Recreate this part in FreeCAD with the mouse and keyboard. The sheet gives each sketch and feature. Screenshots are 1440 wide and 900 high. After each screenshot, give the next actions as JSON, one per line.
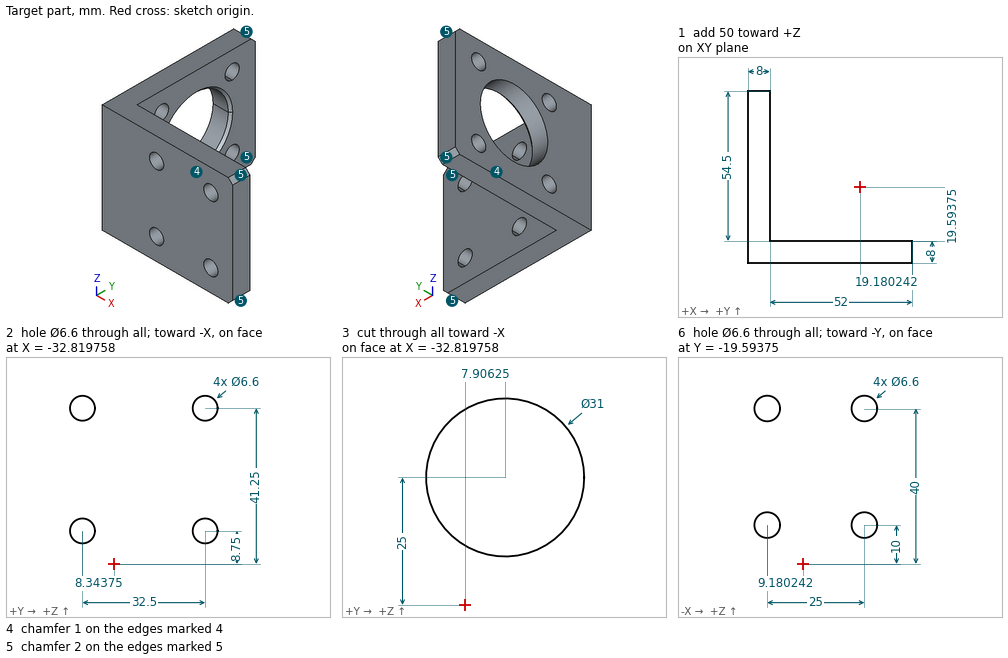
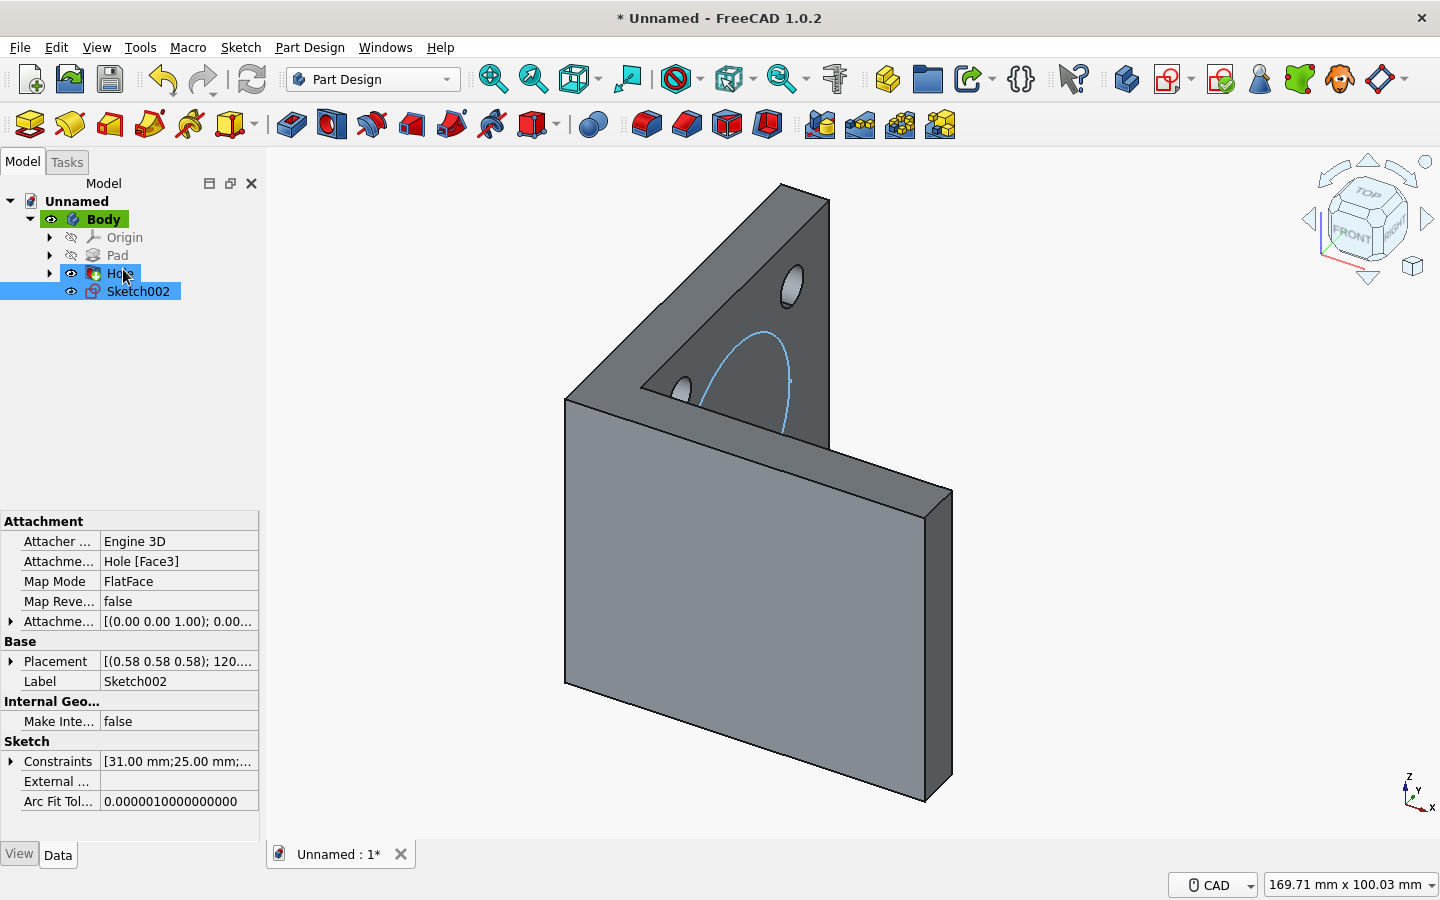
{"action": "left_click", "coordinate": [292, 124]}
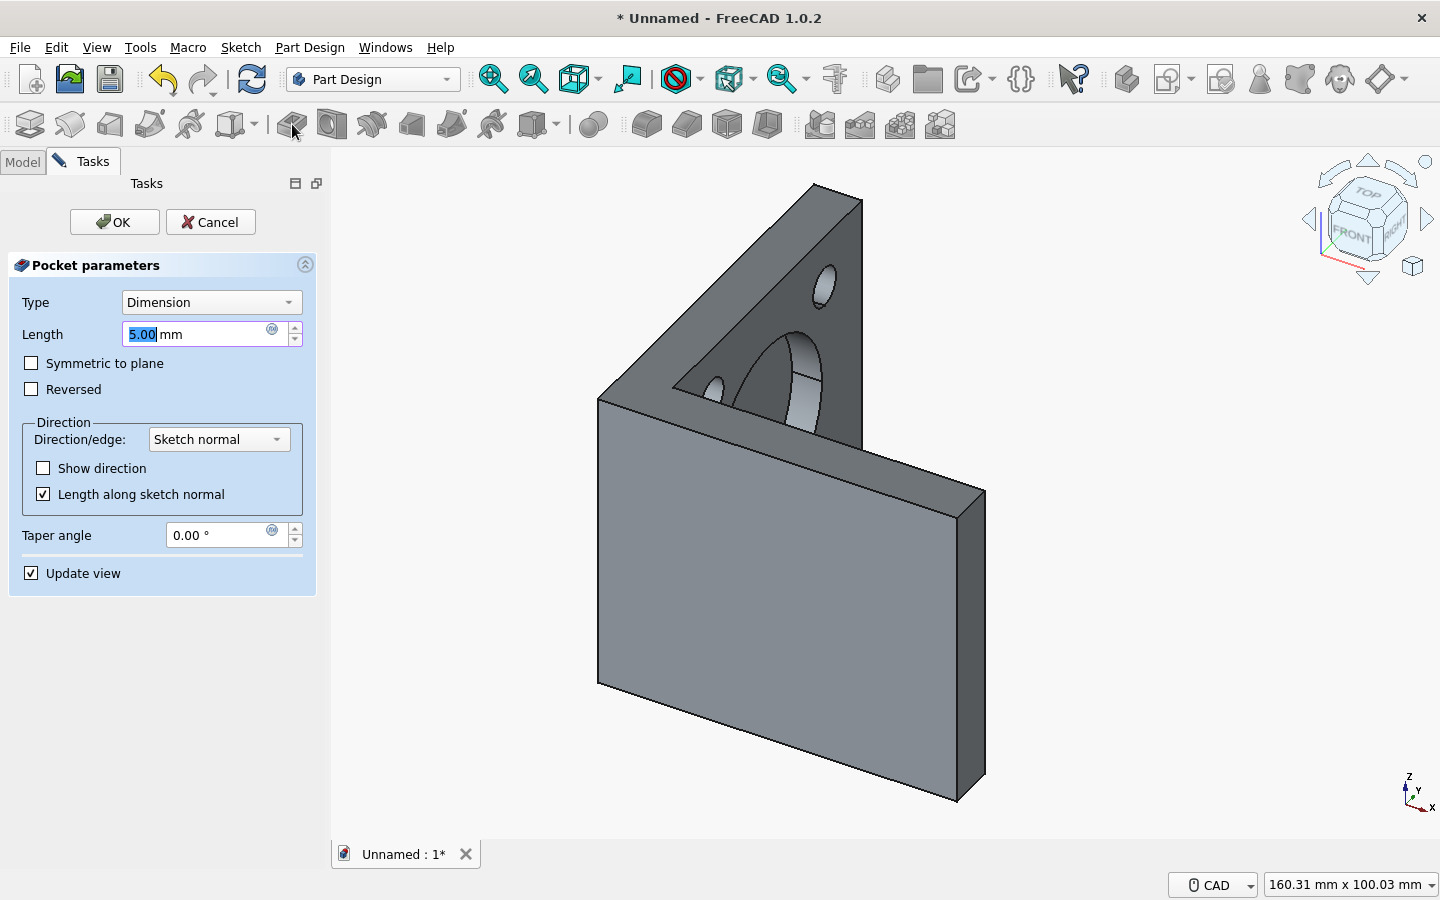
{"action": "left_click", "coordinate": [212, 302]}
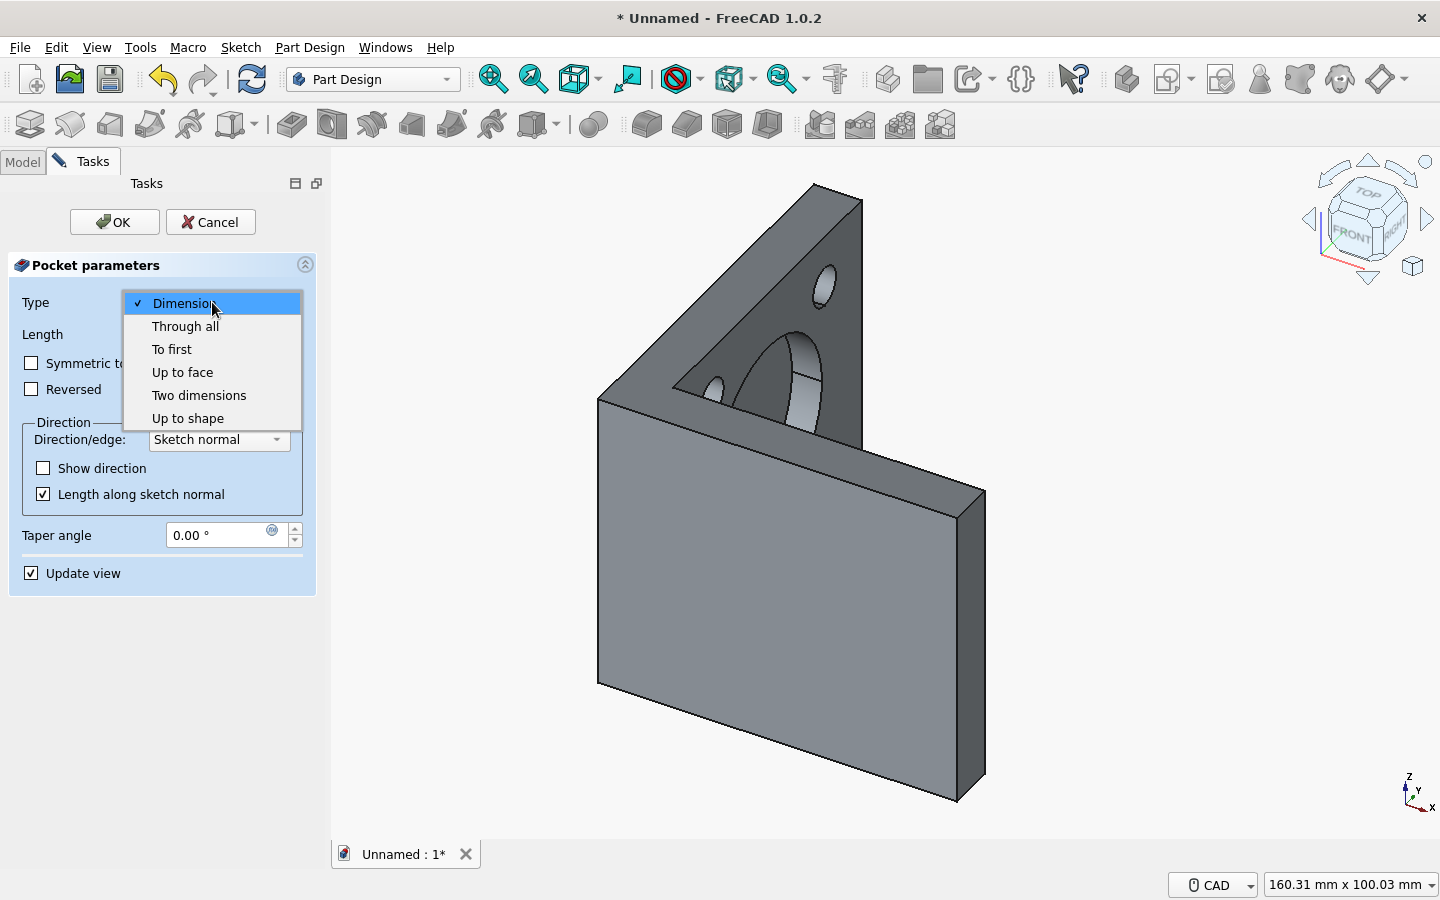
{"action": "left_click", "coordinate": [212, 326]}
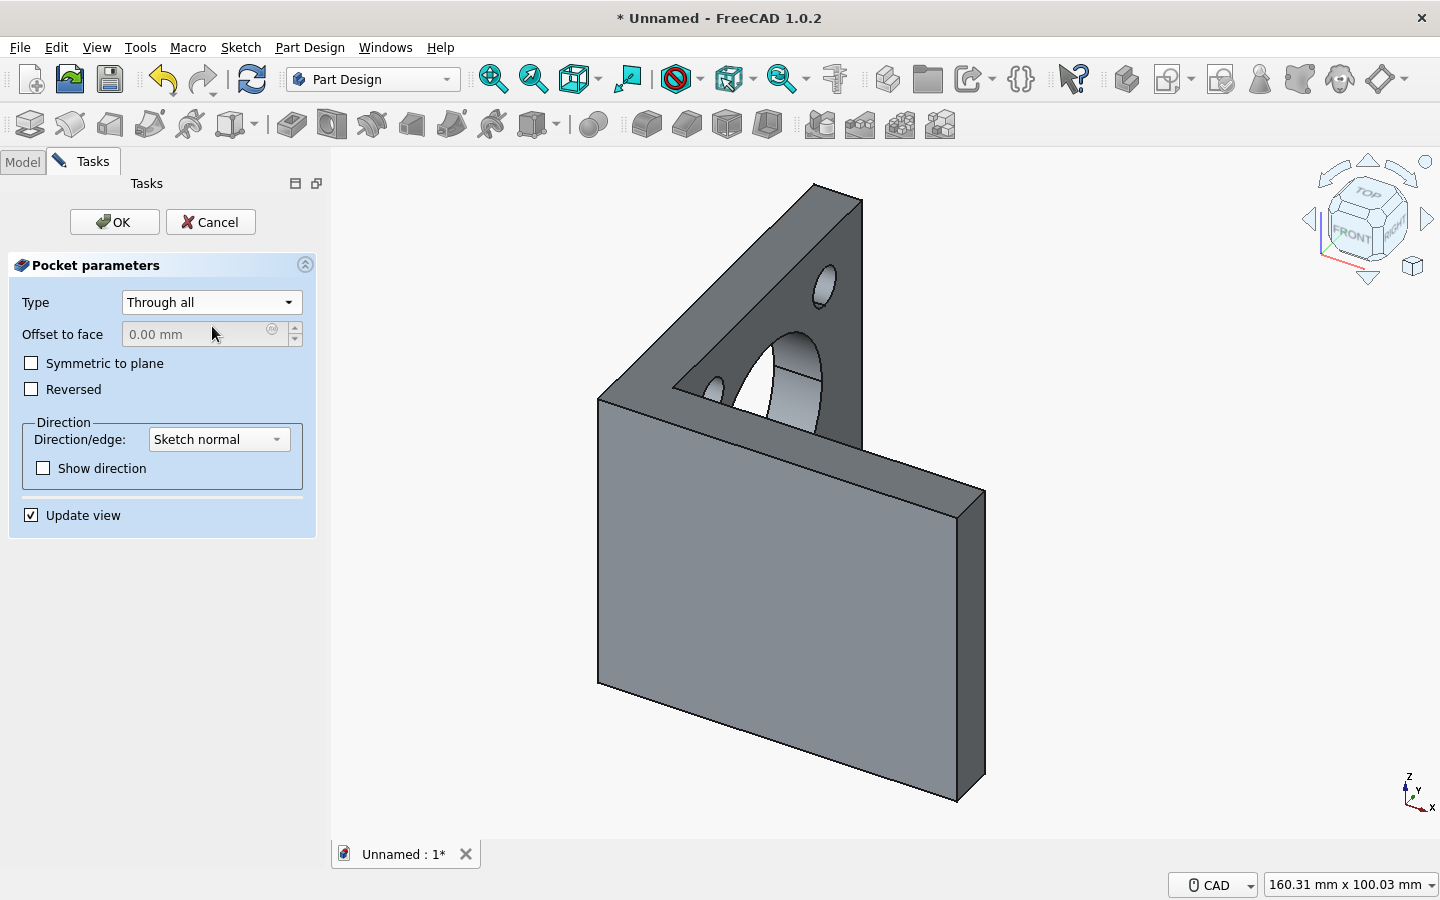
{"action": "left_click", "coordinate": [115, 222]}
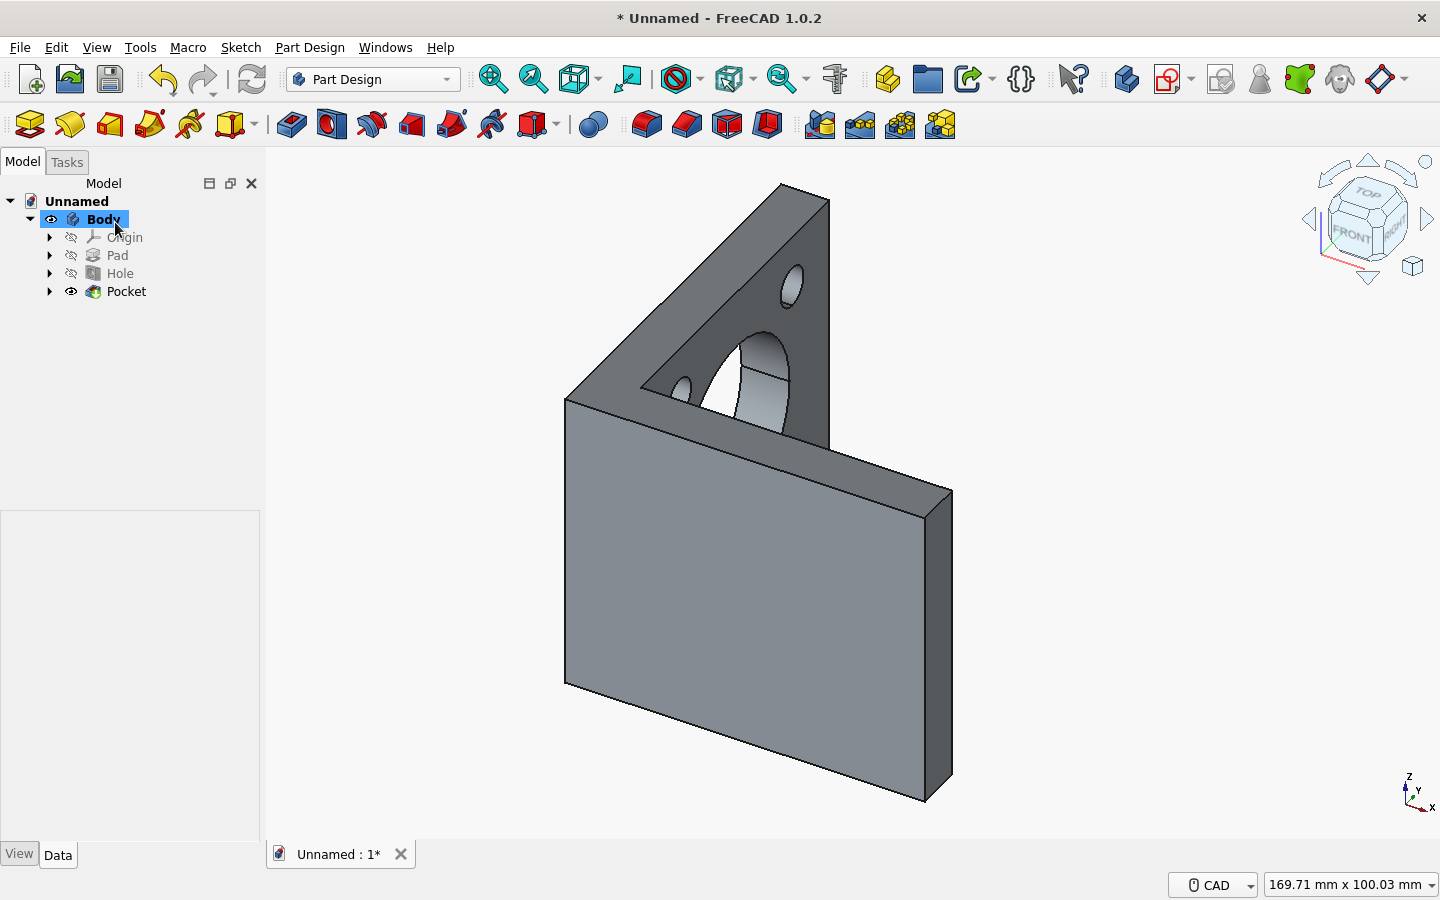
{"action": "left_click", "coordinate": [775, 335]}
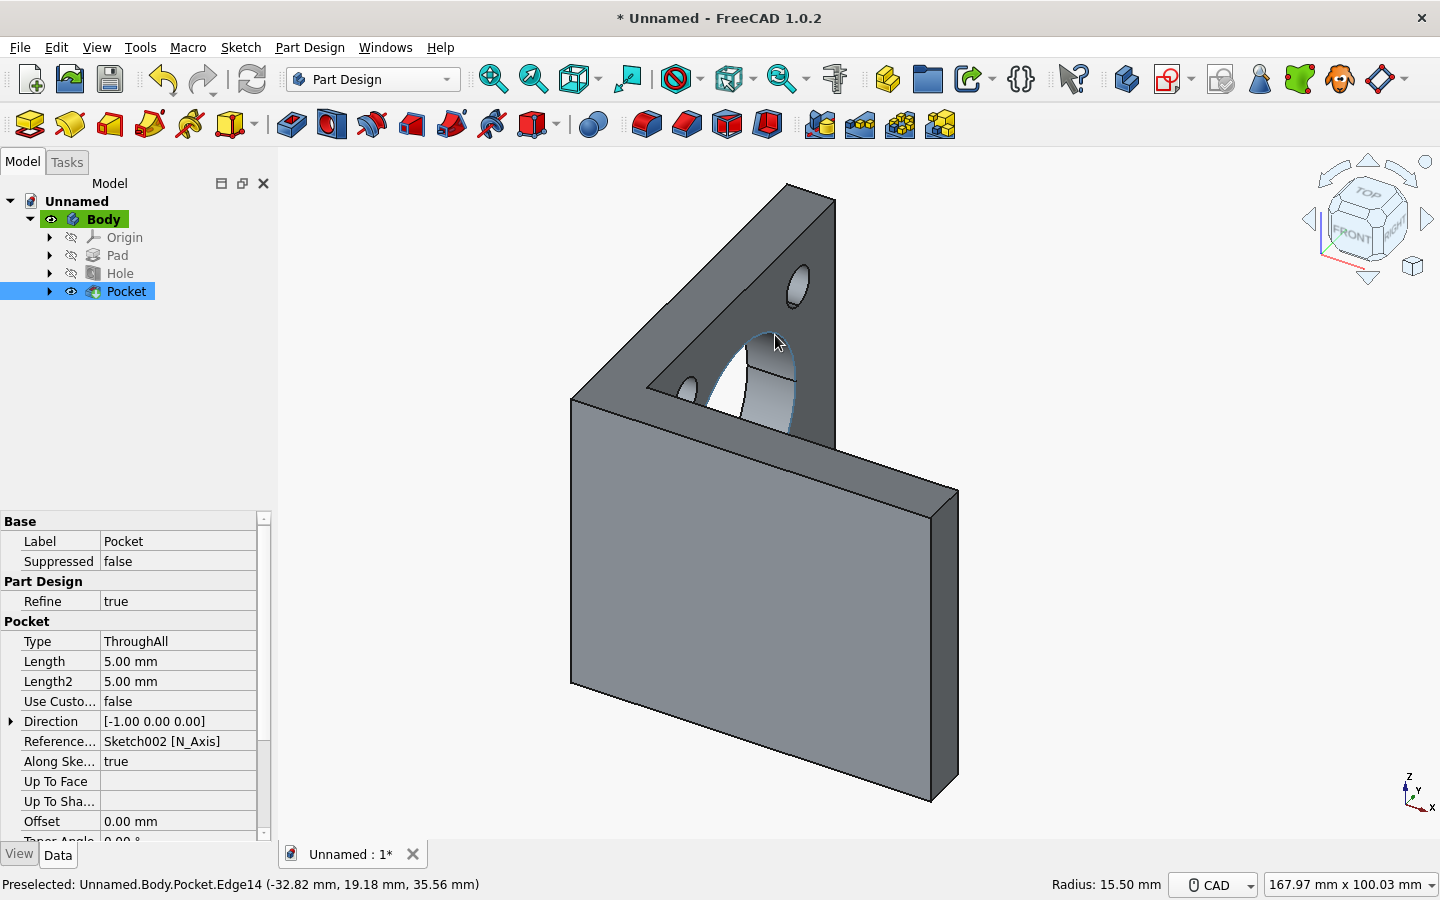
{"action": "left_click", "coordinate": [688, 124]}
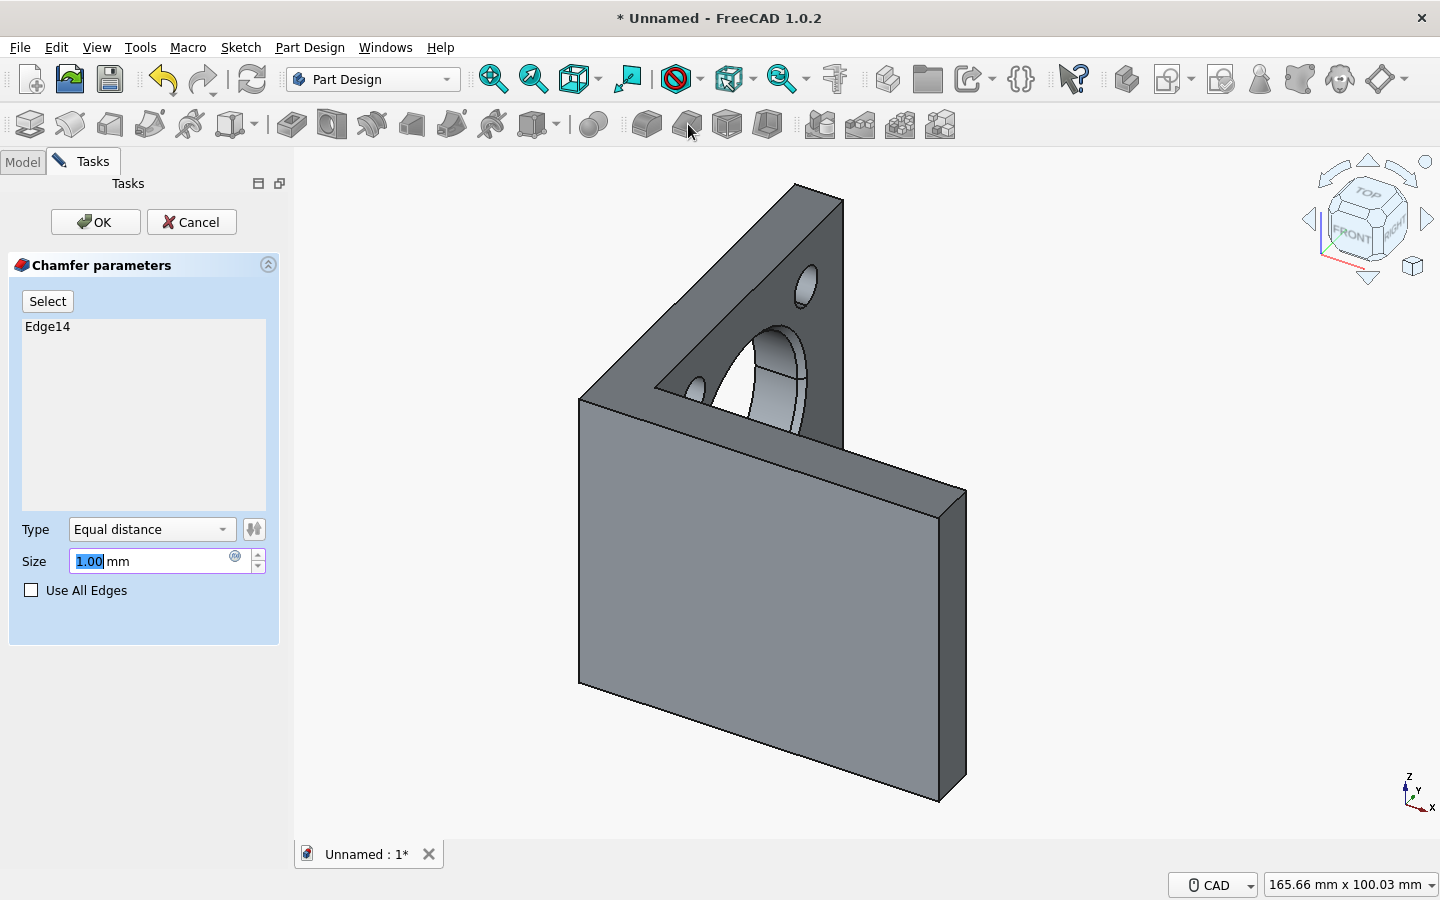
{"action": "type", "text": "1"}
{"action": "key", "text": "Tab"}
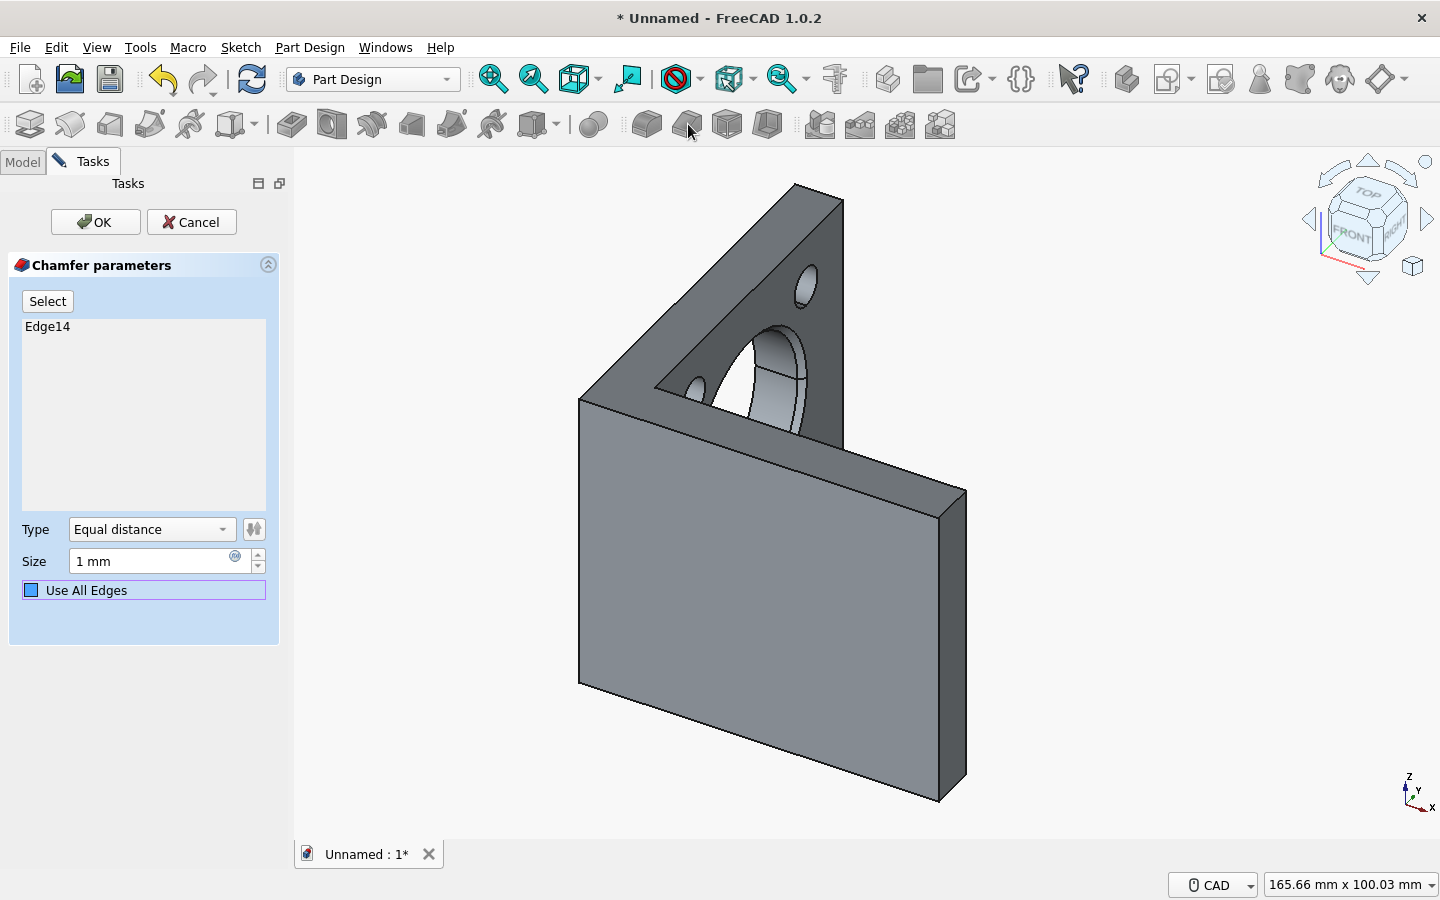
{"action": "left_click", "coordinate": [96, 222]}